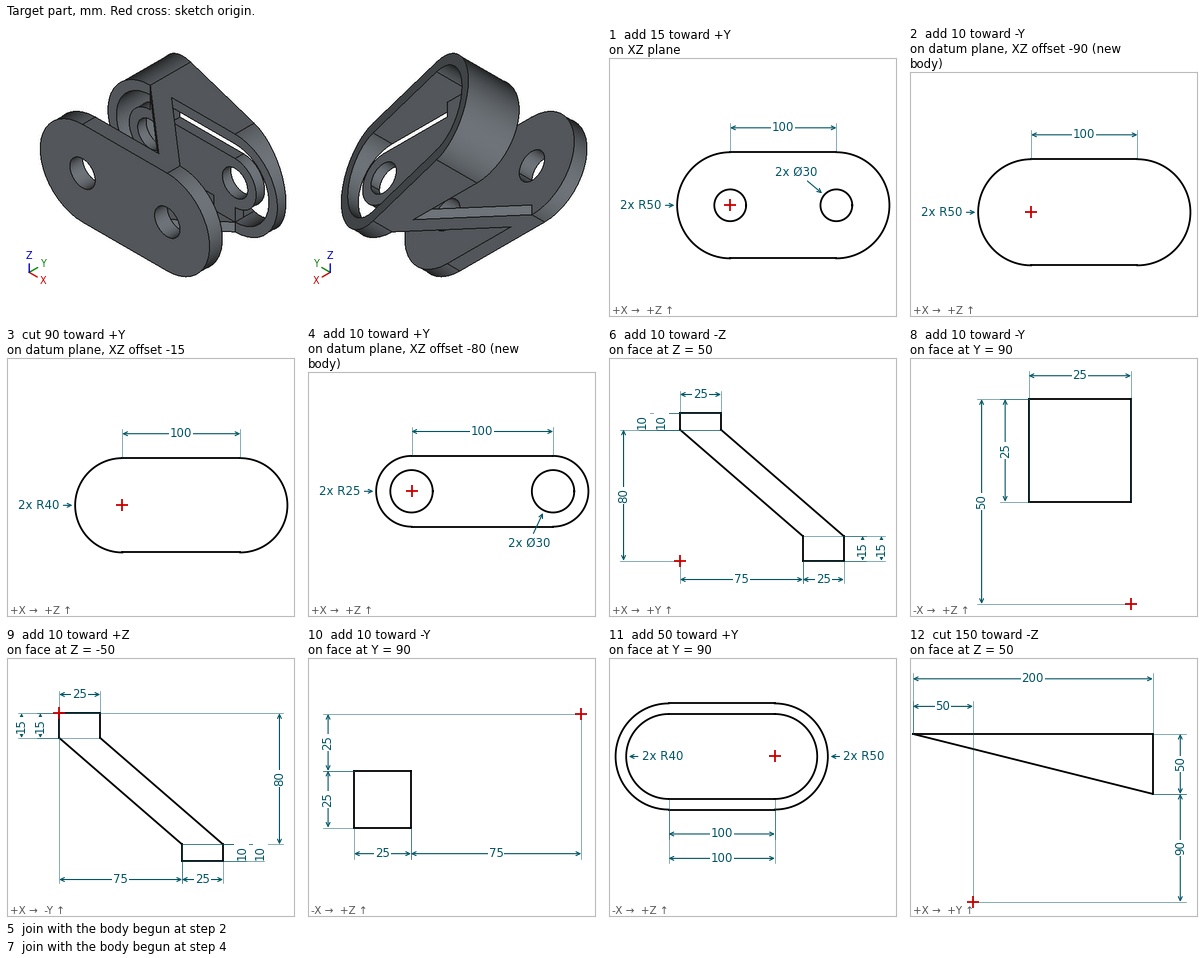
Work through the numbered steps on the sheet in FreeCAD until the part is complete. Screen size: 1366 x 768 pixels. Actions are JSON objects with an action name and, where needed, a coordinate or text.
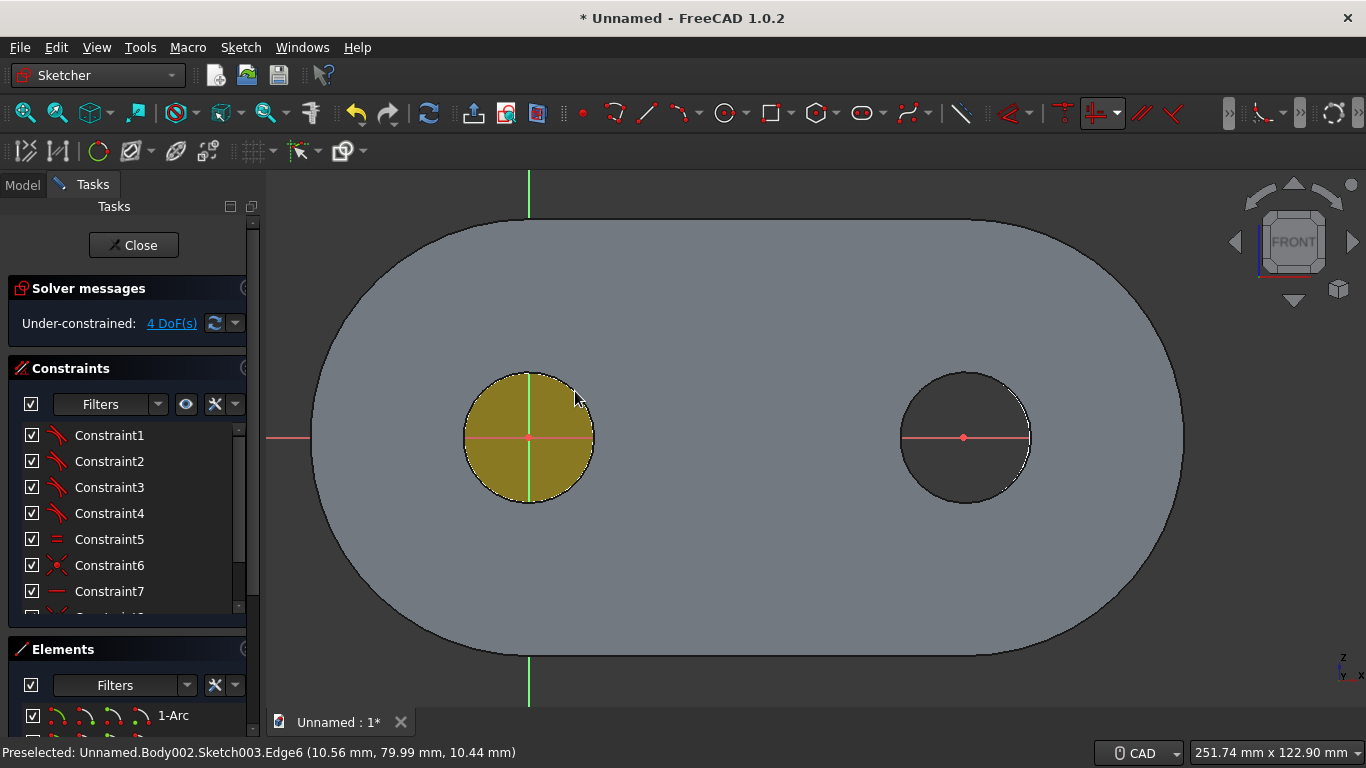
{"action": "left_click", "coordinate": [1011, 391]}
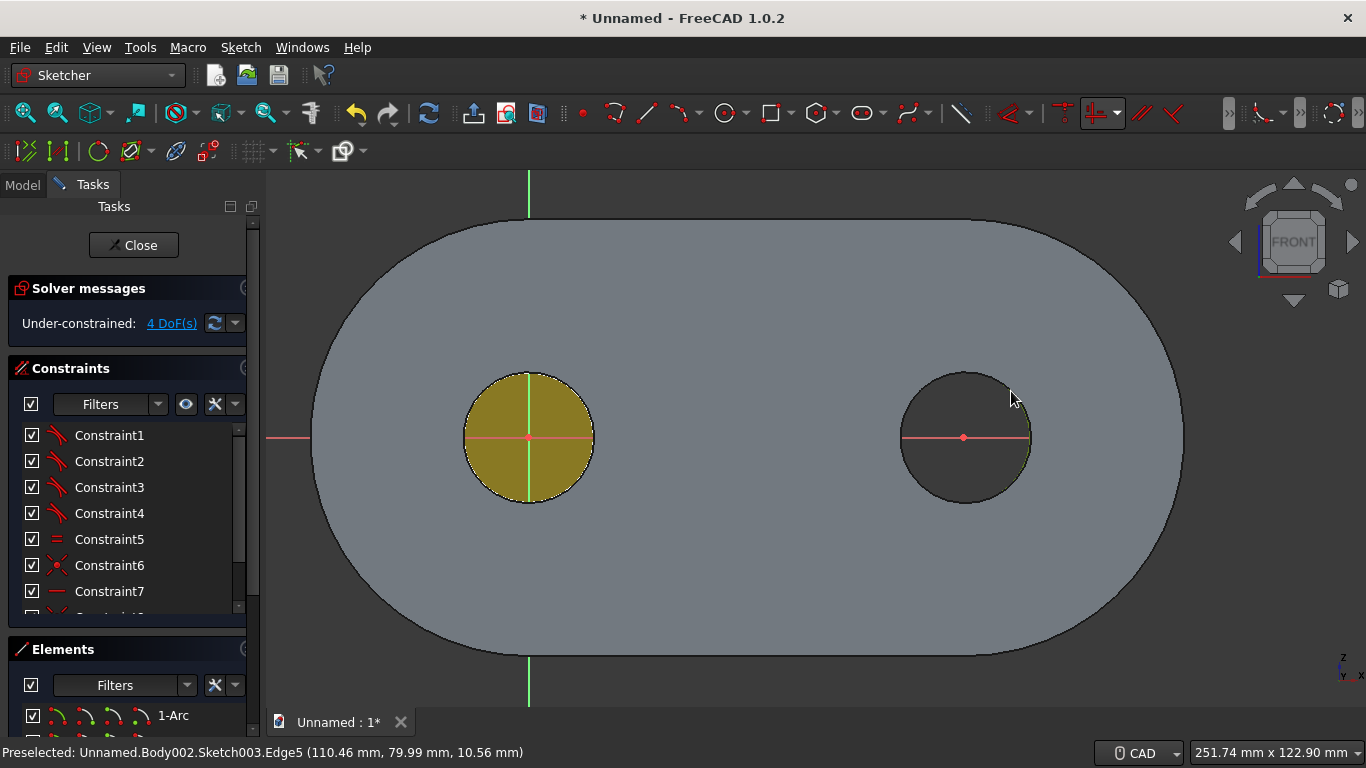
{"action": "left_click", "coordinate": [575, 392]}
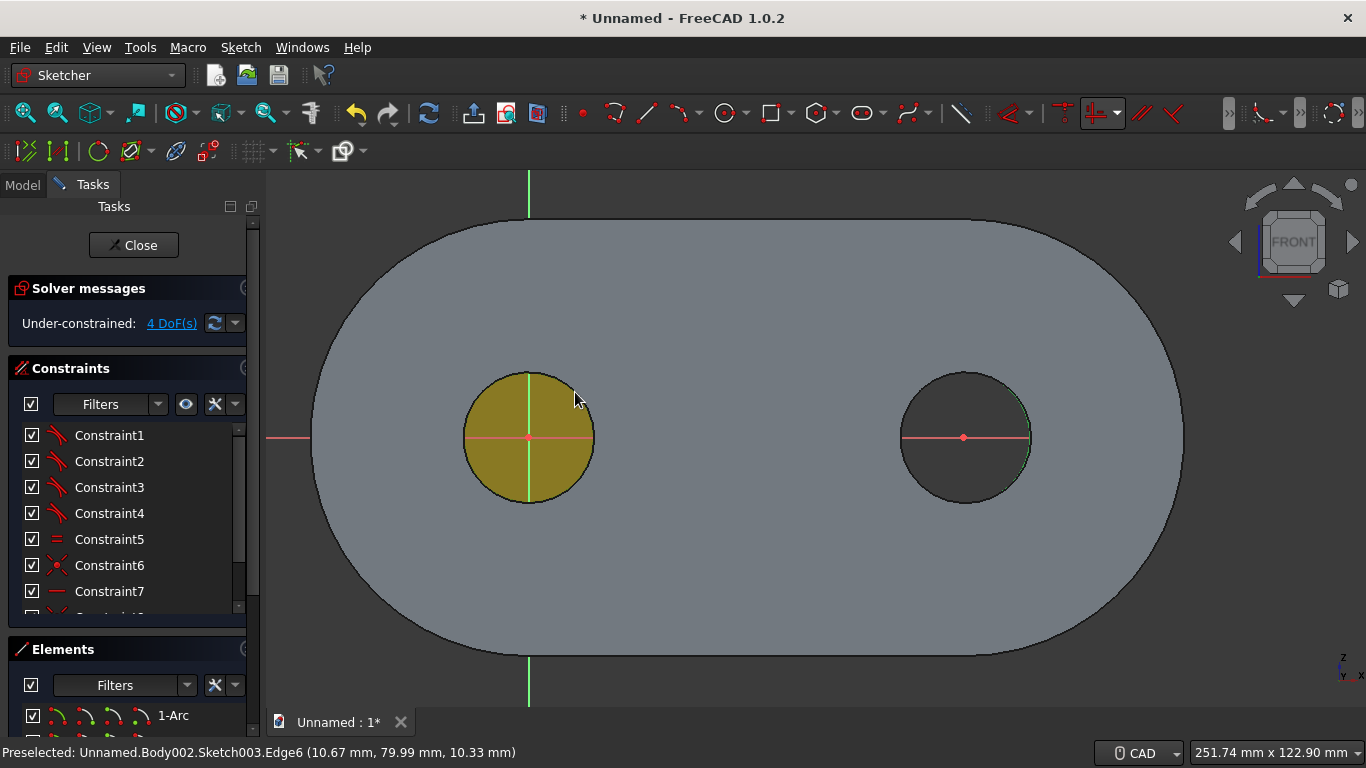
{"action": "key", "text": "e"}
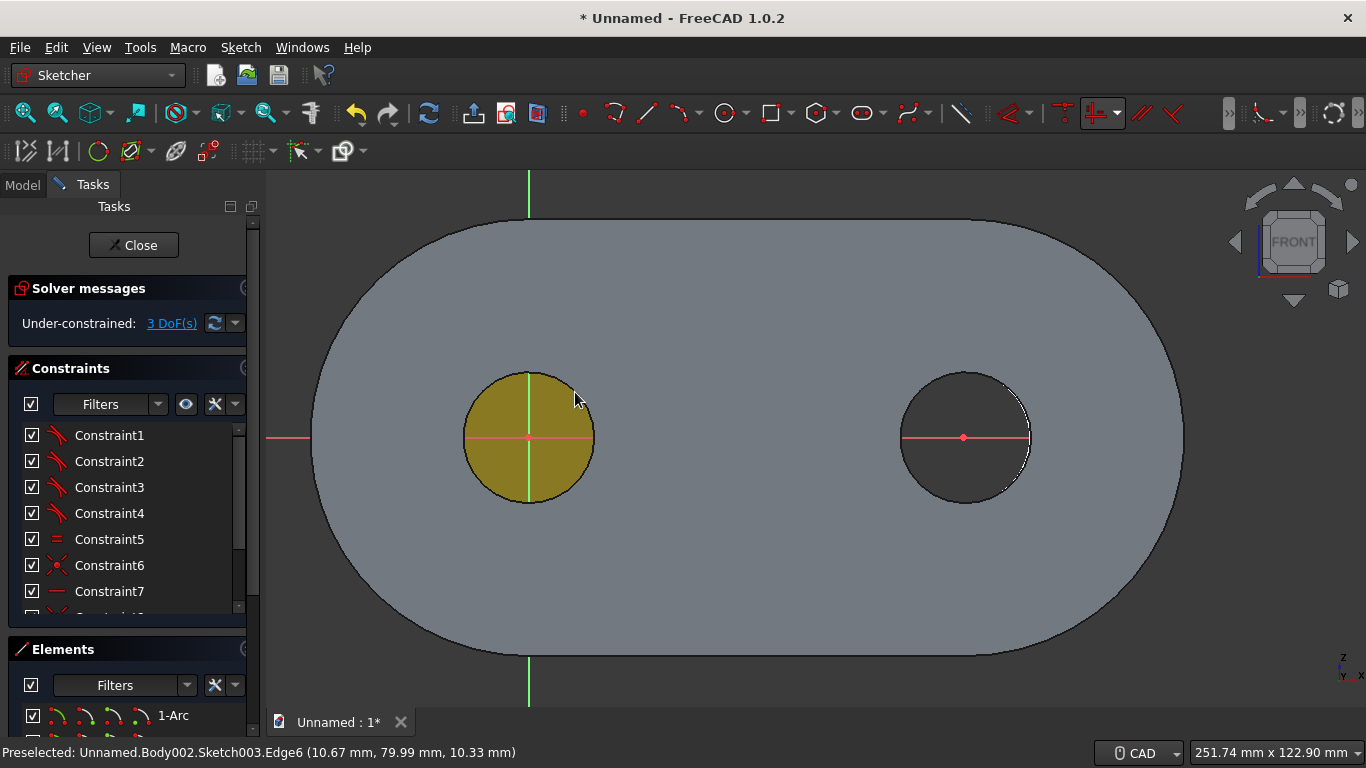
{"action": "left_click", "coordinate": [1008, 114]}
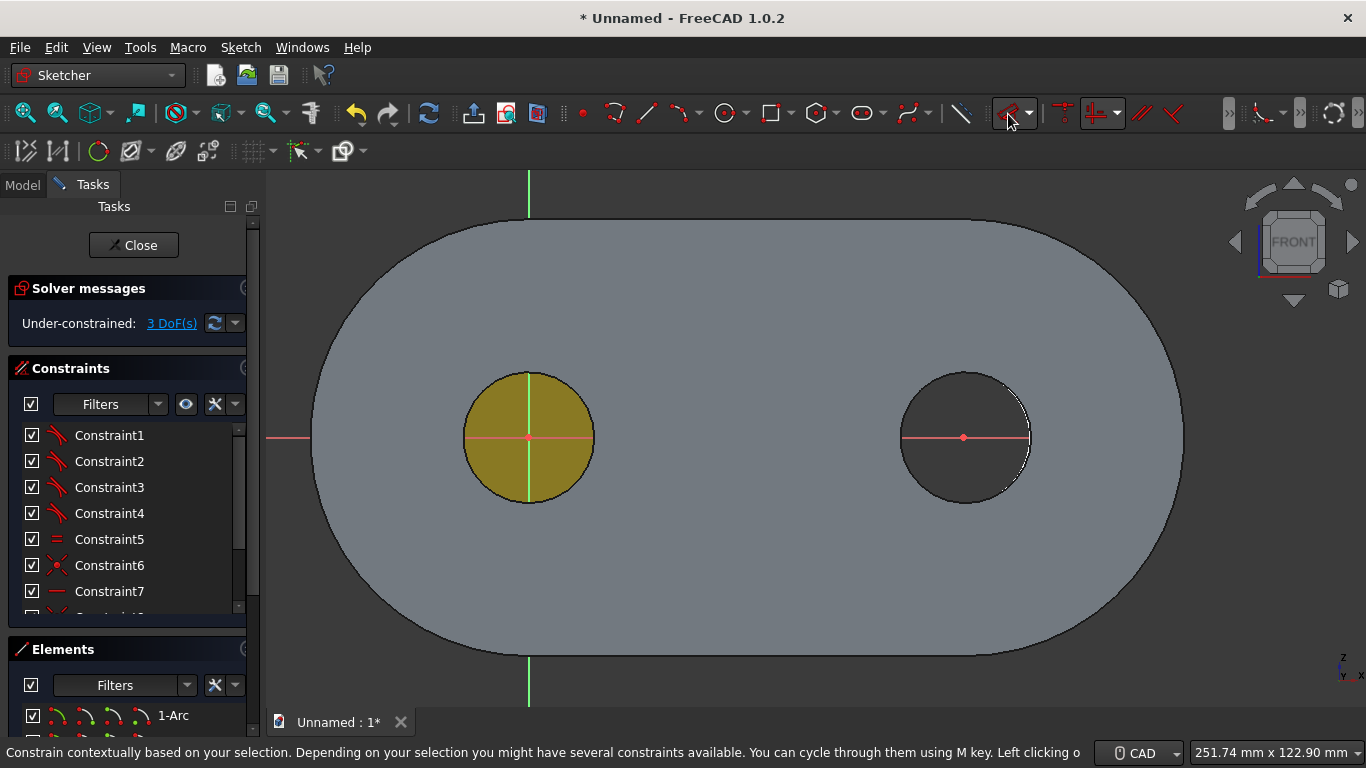
{"action": "left_click", "coordinate": [443, 375]}
{"action": "left_click", "coordinate": [417, 356]}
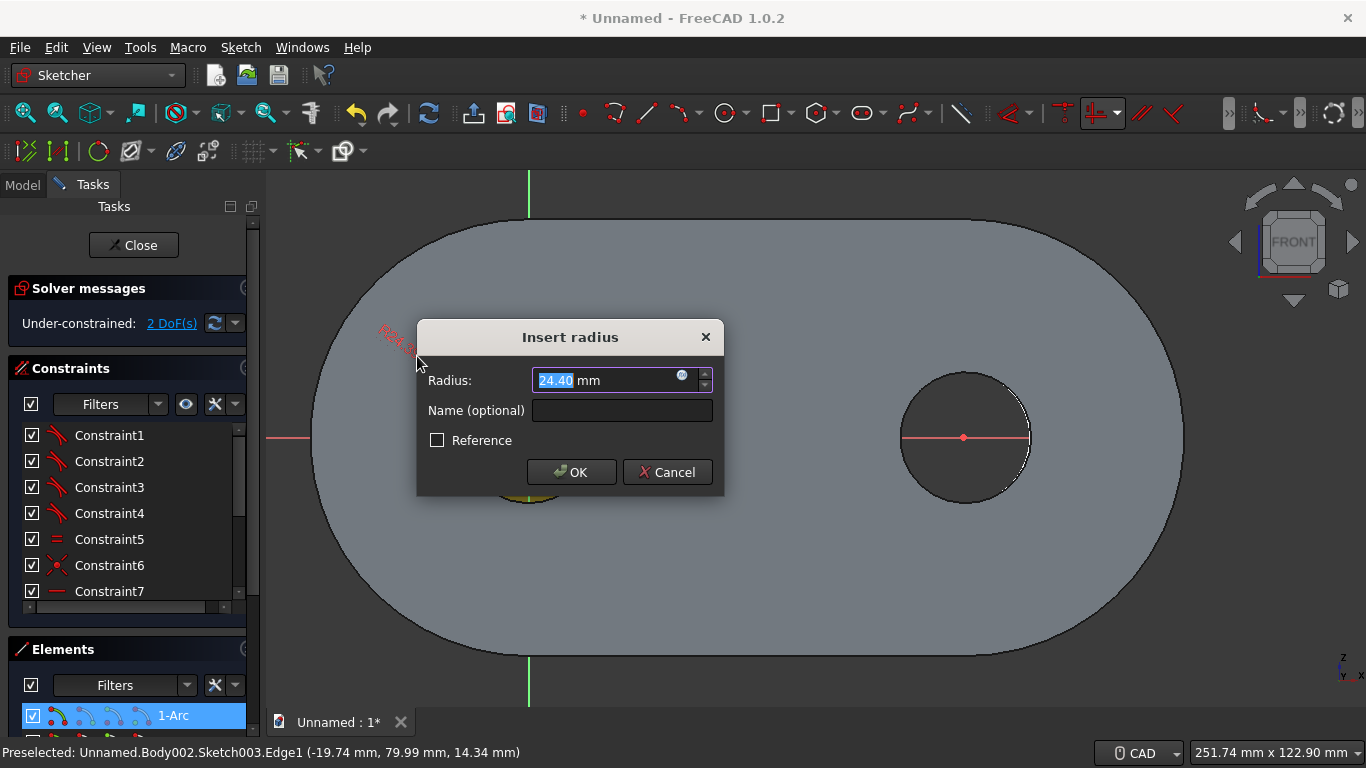
{"action": "type", "text": "25"}
{"action": "key", "text": "Return"}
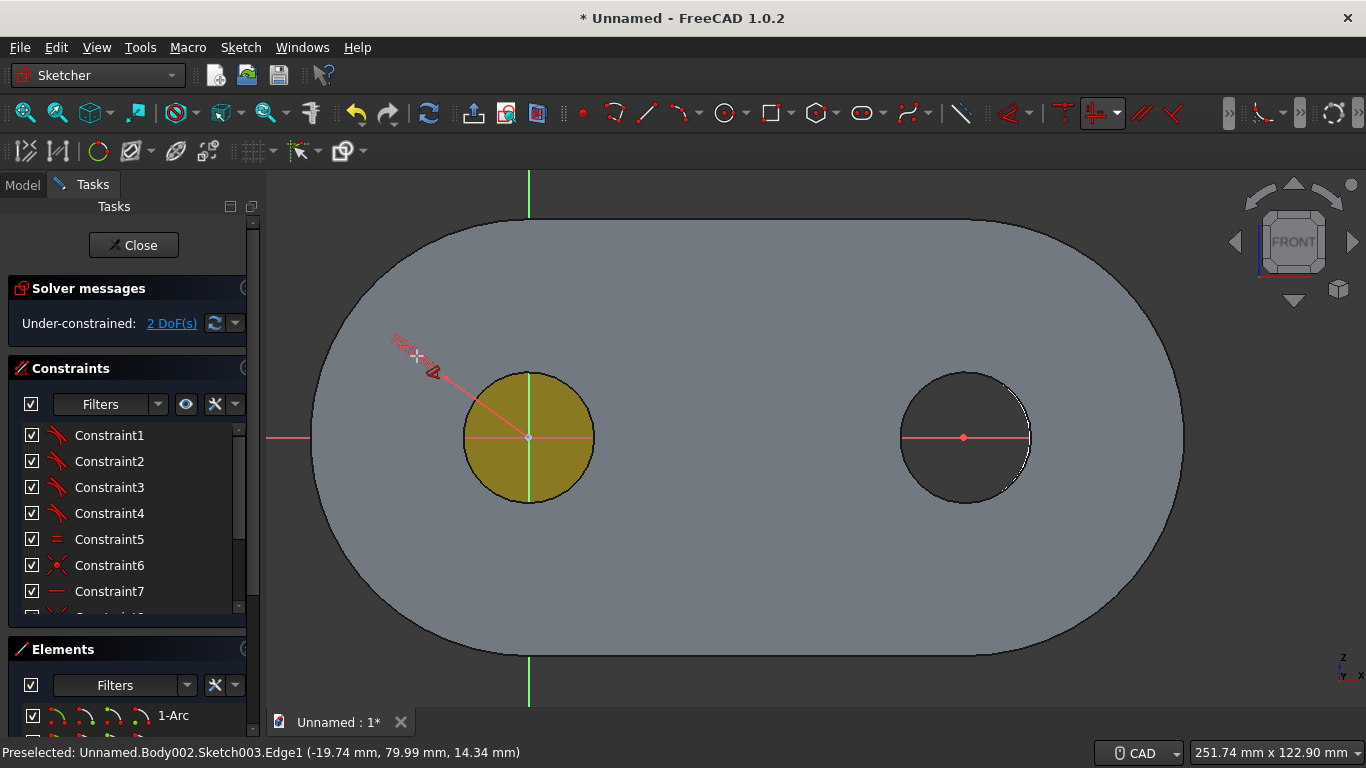
{"action": "left_click", "coordinate": [1011, 391]}
{"action": "left_click", "coordinate": [943, 342]}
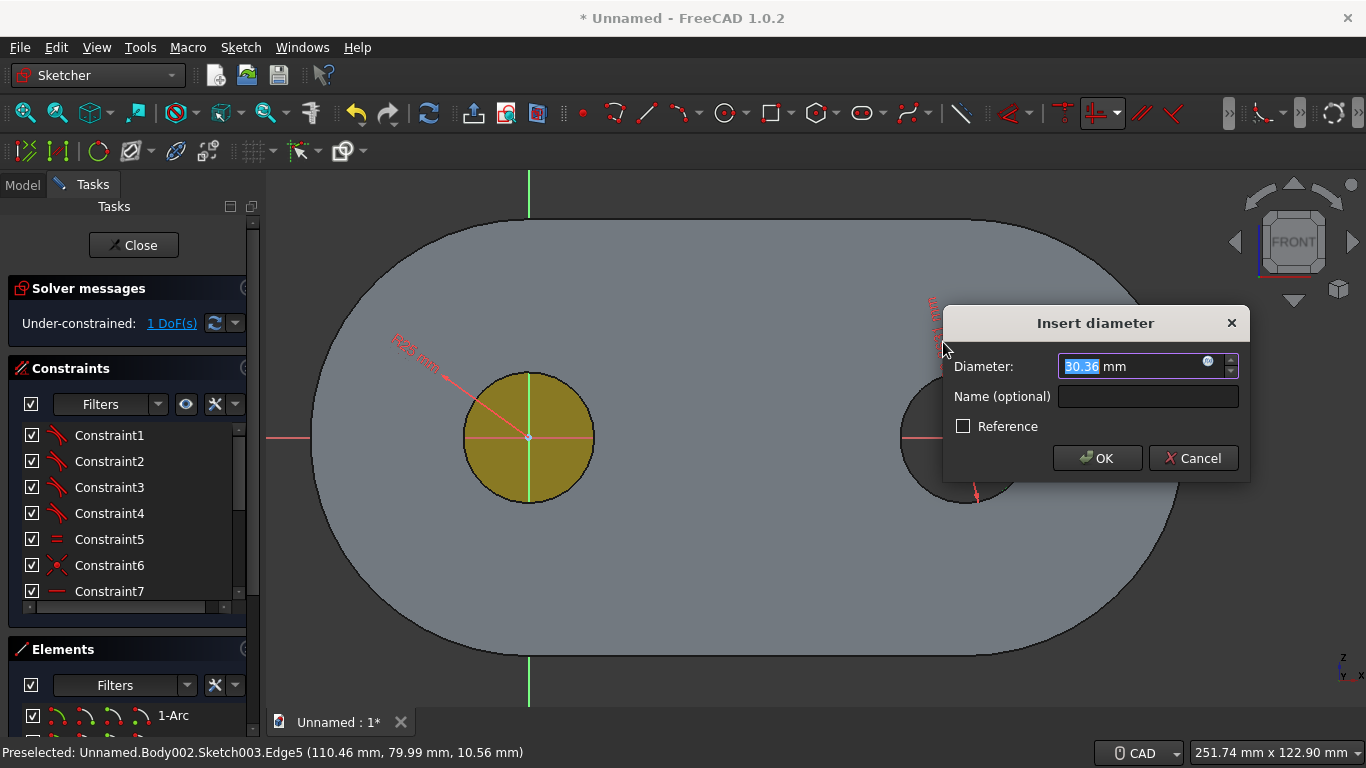
{"action": "type", "text": "30"}
{"action": "key", "text": "Return"}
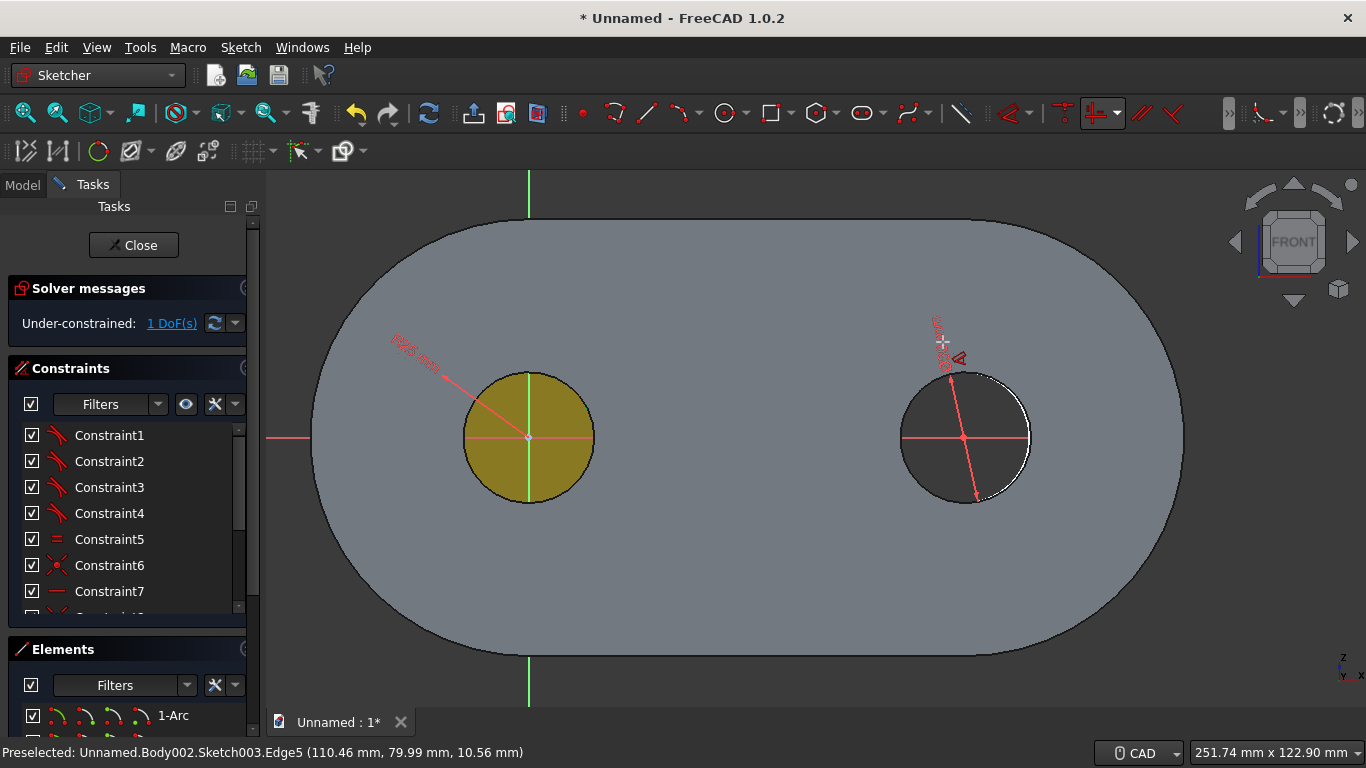
{"action": "left_click", "coordinate": [659, 328]}
{"action": "left_click", "coordinate": [746, 294]}